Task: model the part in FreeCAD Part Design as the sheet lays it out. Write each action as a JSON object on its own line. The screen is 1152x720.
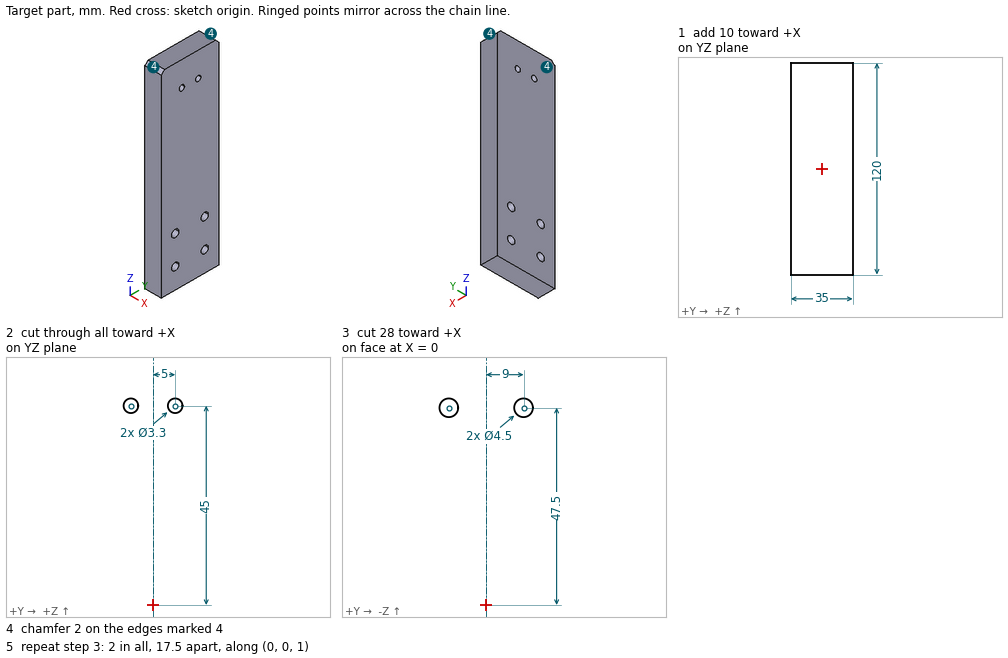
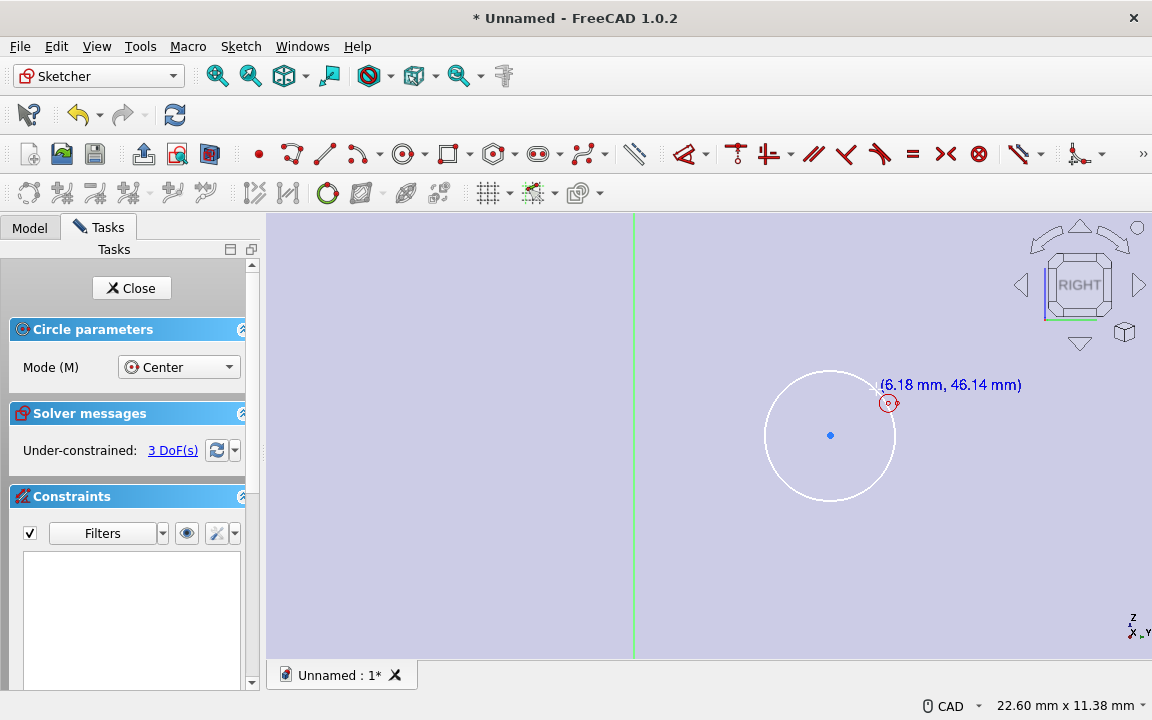
{"action": "left_click", "coordinate": [438, 435]}
{"action": "left_click", "coordinate": [483, 389]}
{"action": "key", "text": "Escape"}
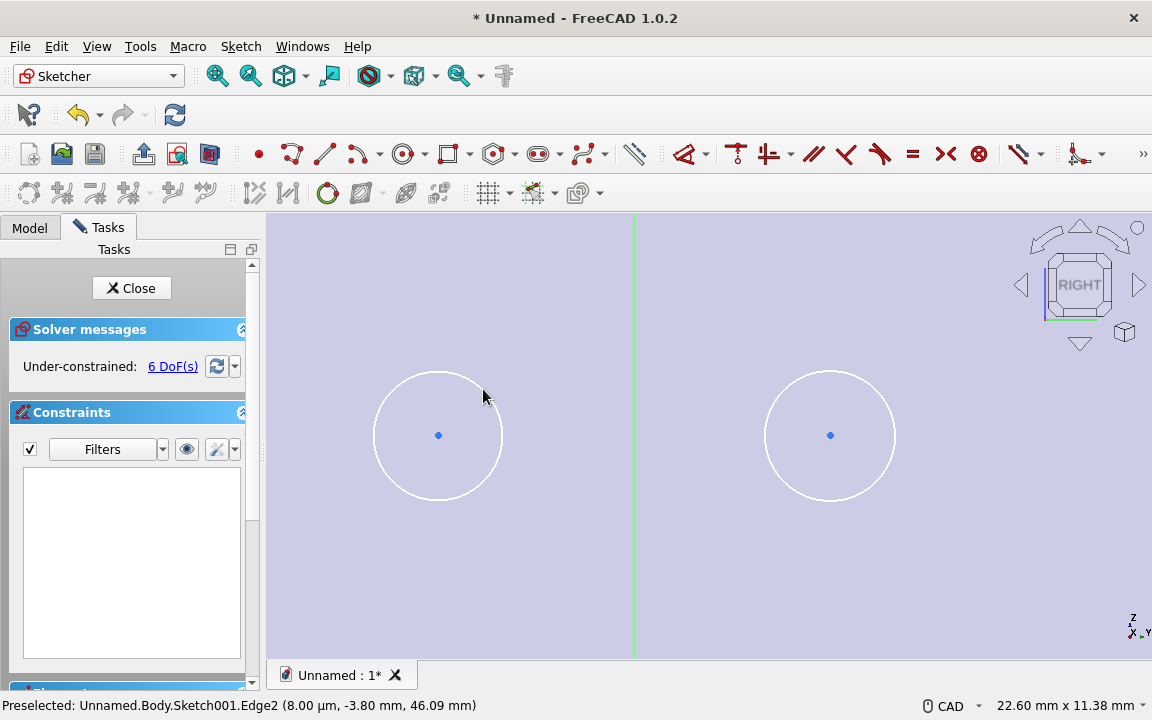
{"action": "left_click", "coordinate": [876, 390]}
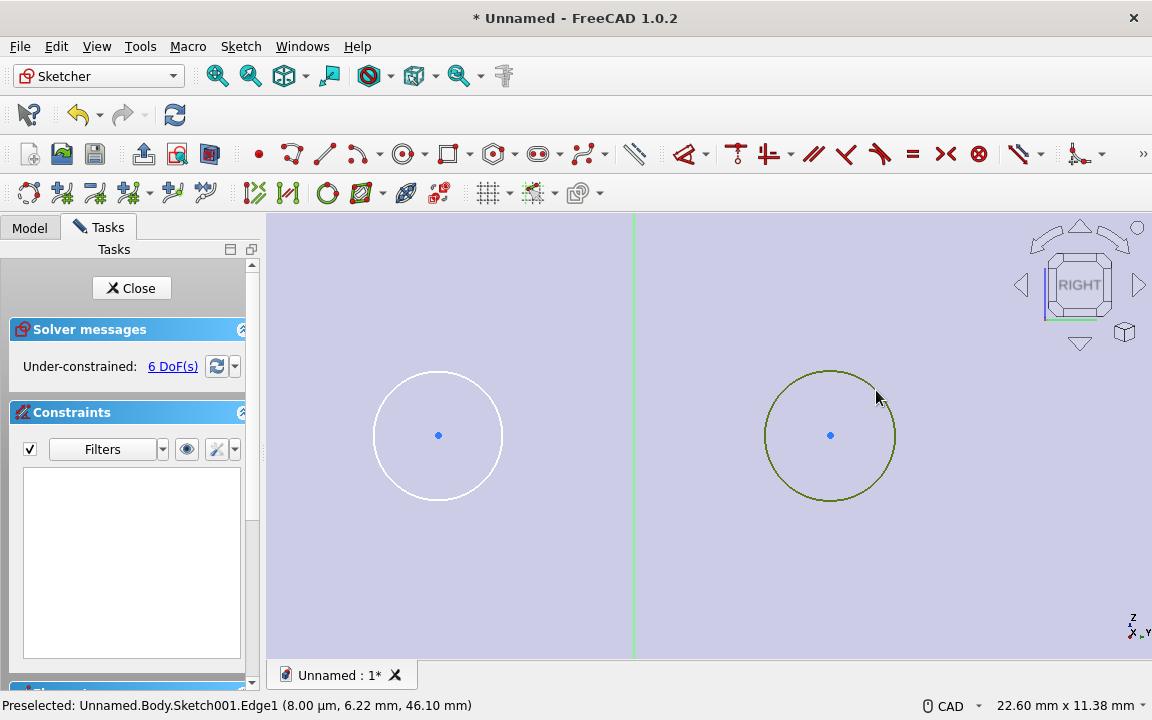
{"action": "left_click", "coordinate": [483, 390]}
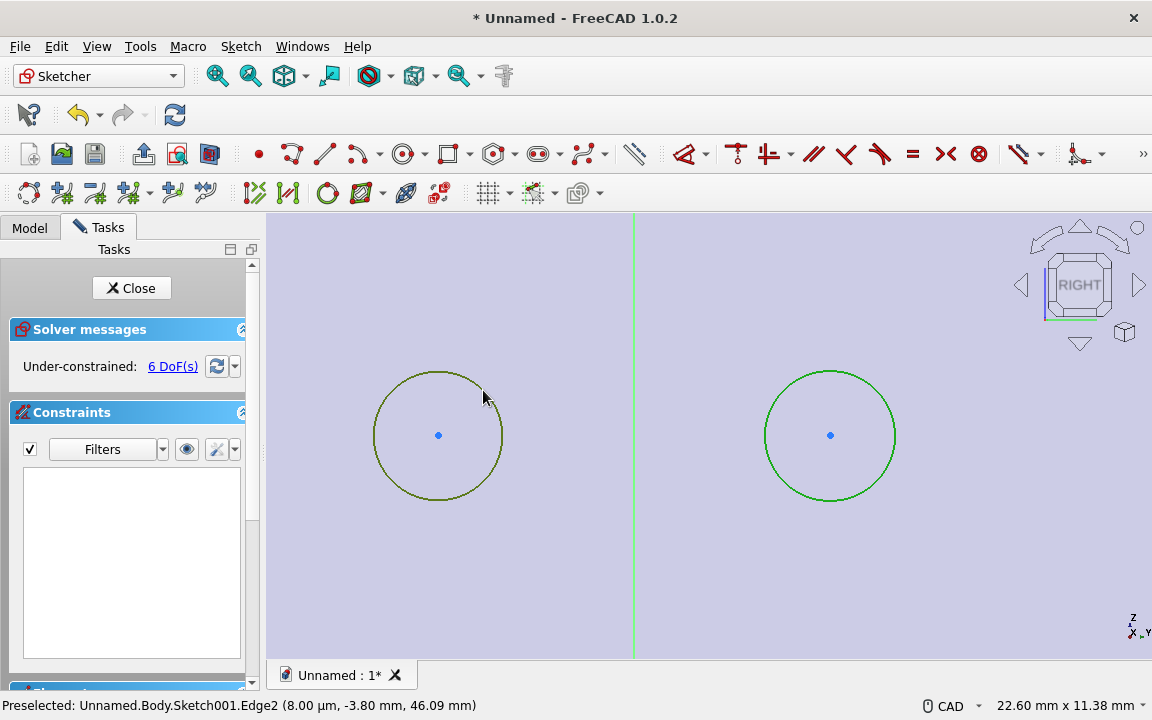
{"action": "left_click", "coordinate": [913, 154]}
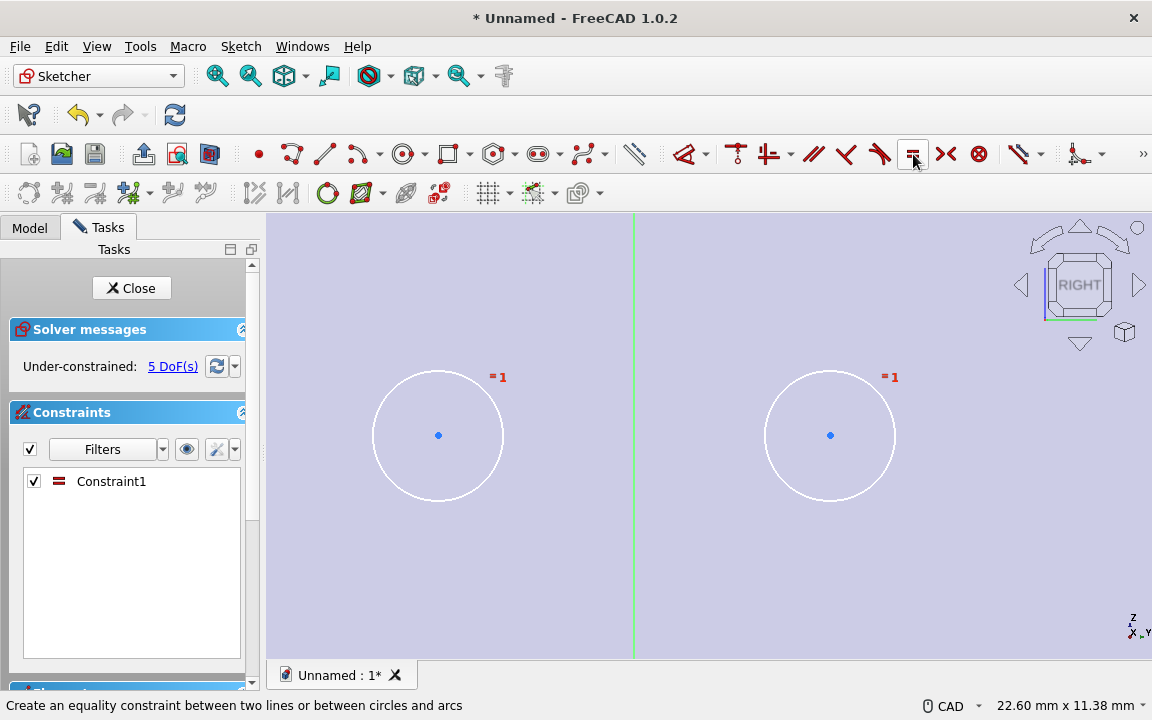
{"action": "left_click", "coordinate": [830, 436]}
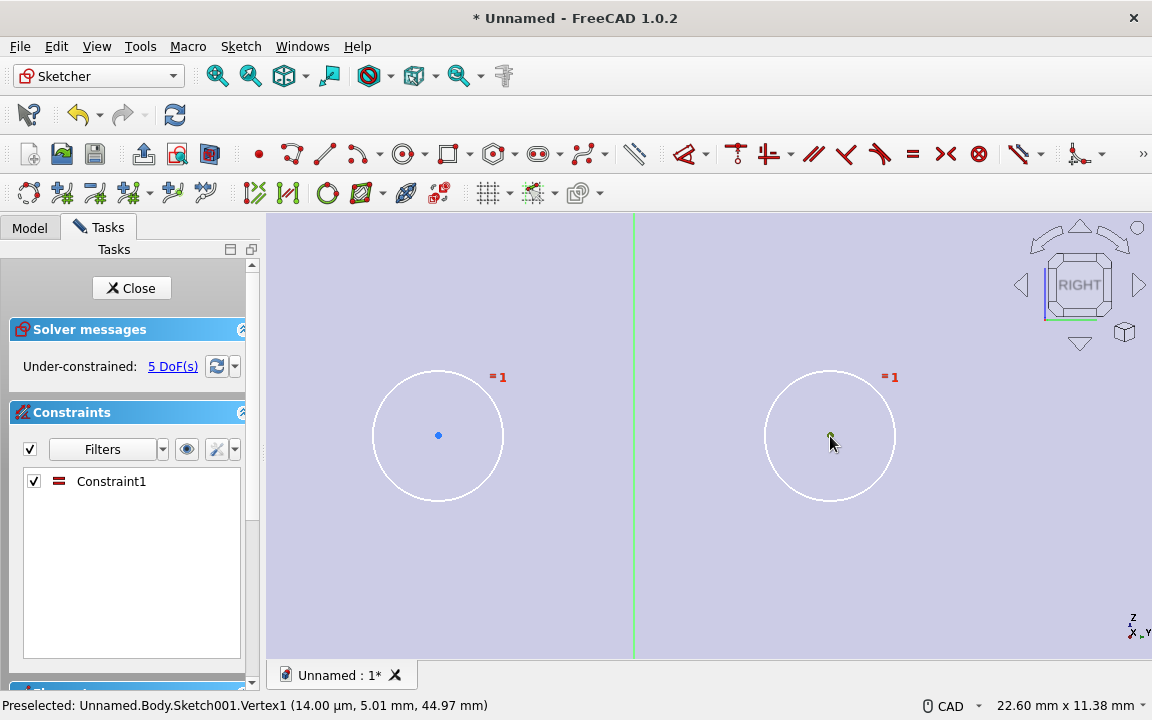
{"action": "left_click", "coordinate": [438, 436]}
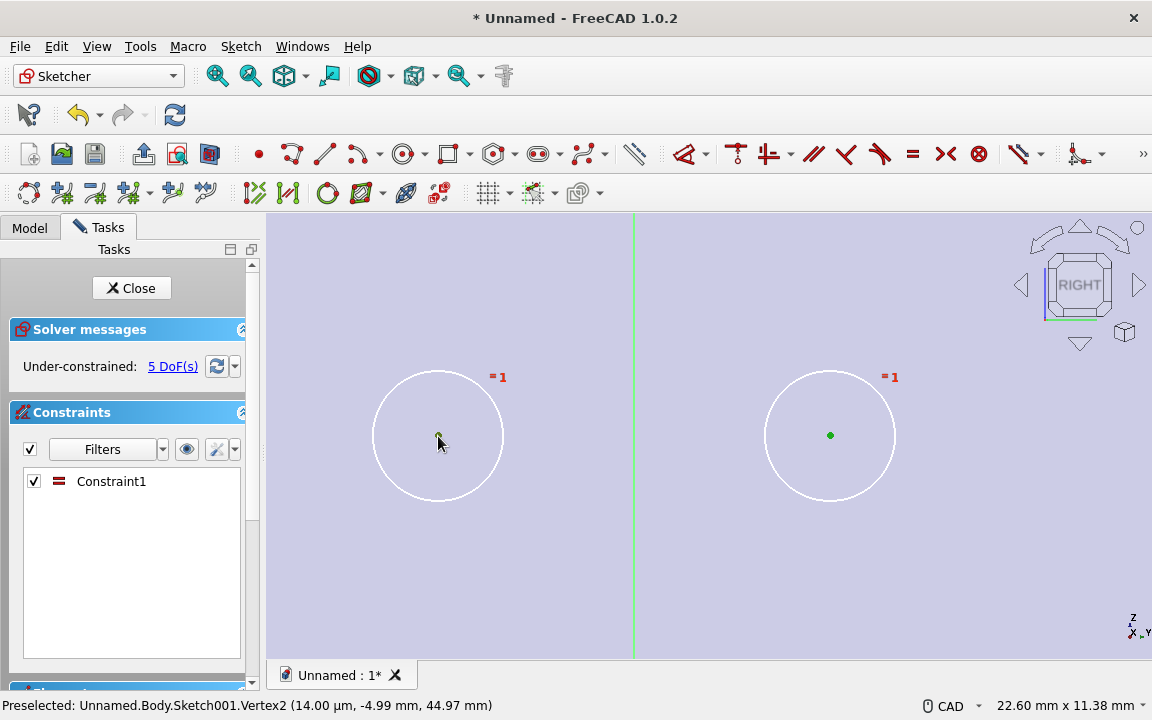
{"action": "left_click", "coordinate": [634, 603]}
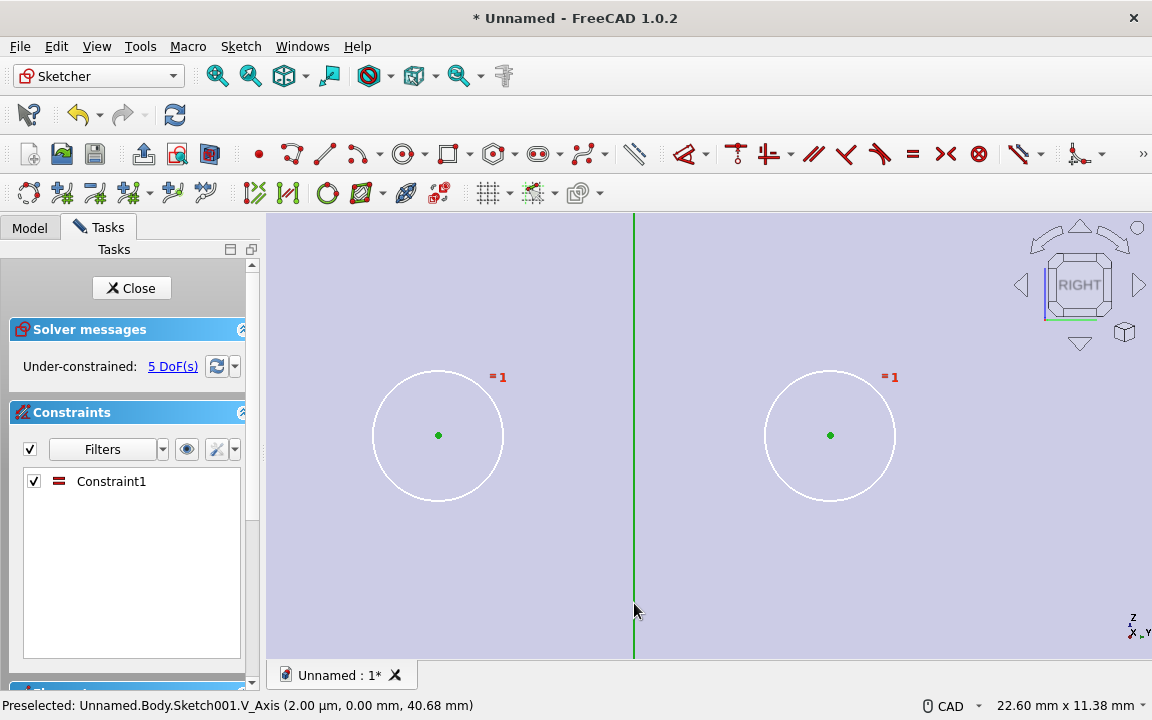
{"action": "left_click", "coordinate": [946, 154]}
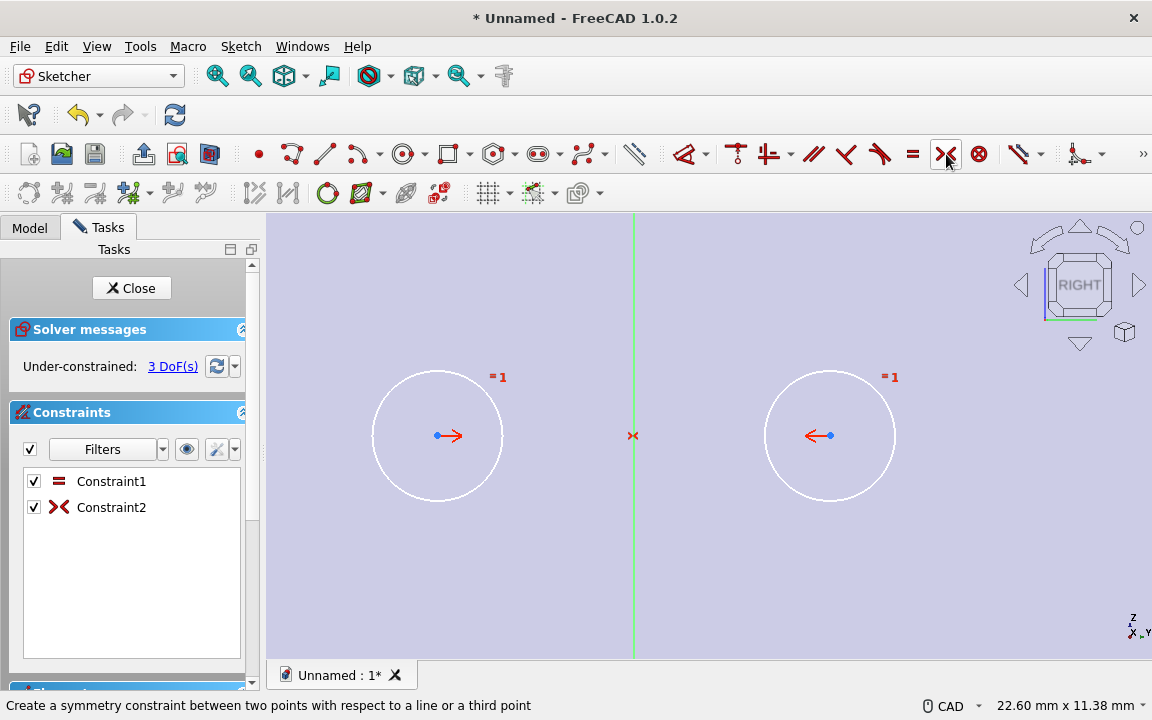
{"action": "left_click", "coordinate": [684, 154]}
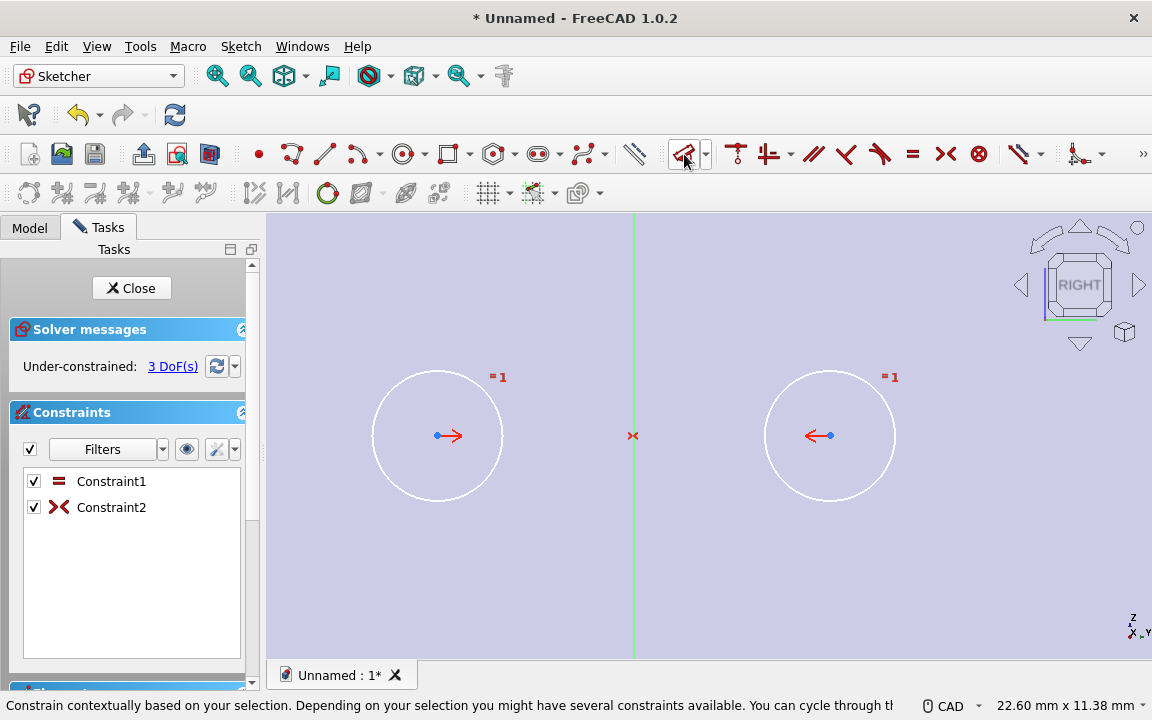
{"action": "left_click", "coordinate": [876, 390]}
{"action": "left_click", "coordinate": [899, 367]}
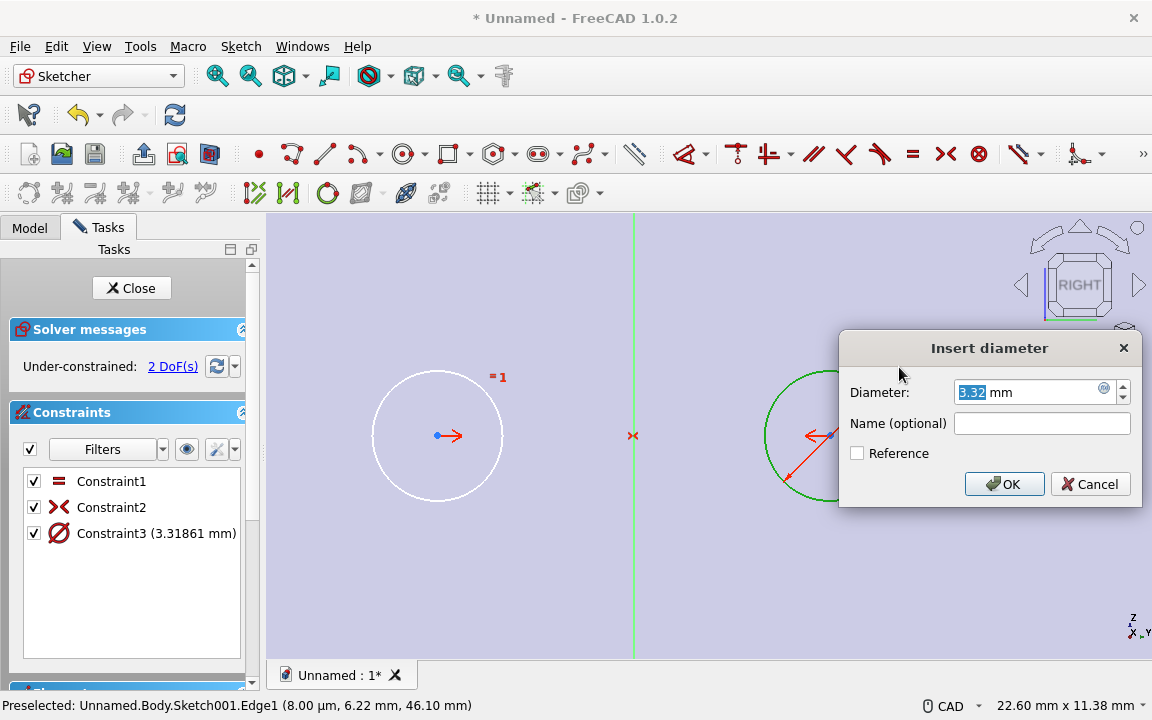
{"action": "type", "text": "3.3"}
{"action": "key", "text": "Return"}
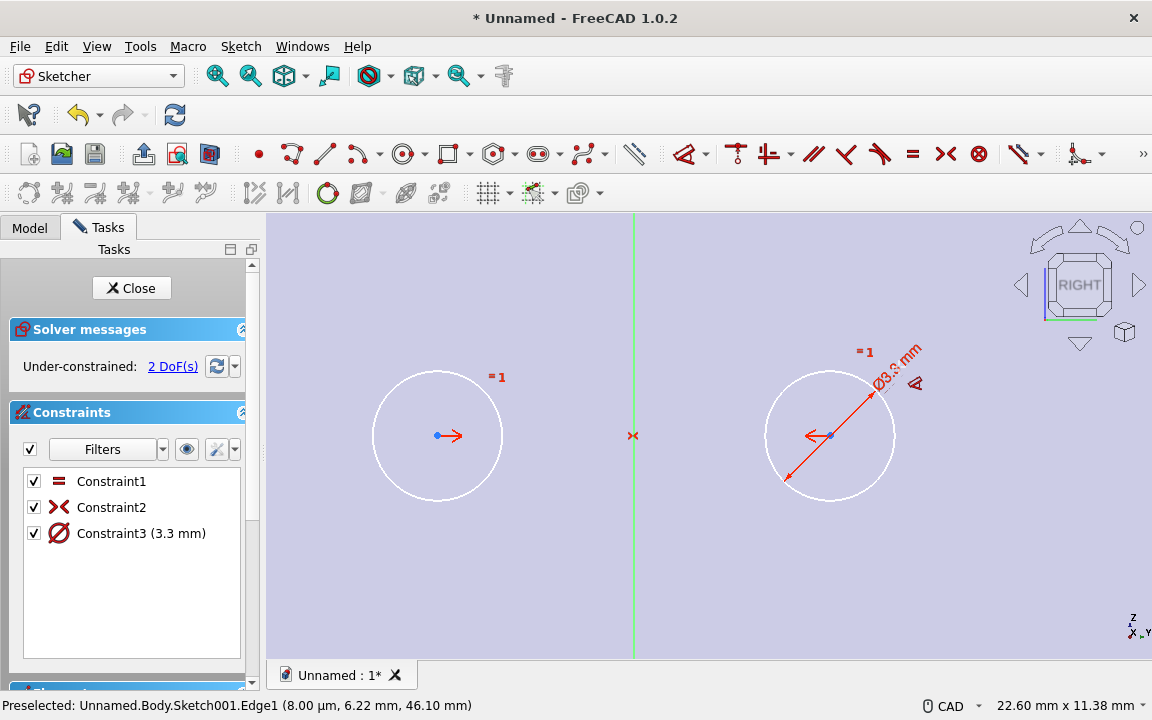
{"action": "left_click", "coordinate": [830, 436]}
{"action": "left_click", "coordinate": [732, 402]}